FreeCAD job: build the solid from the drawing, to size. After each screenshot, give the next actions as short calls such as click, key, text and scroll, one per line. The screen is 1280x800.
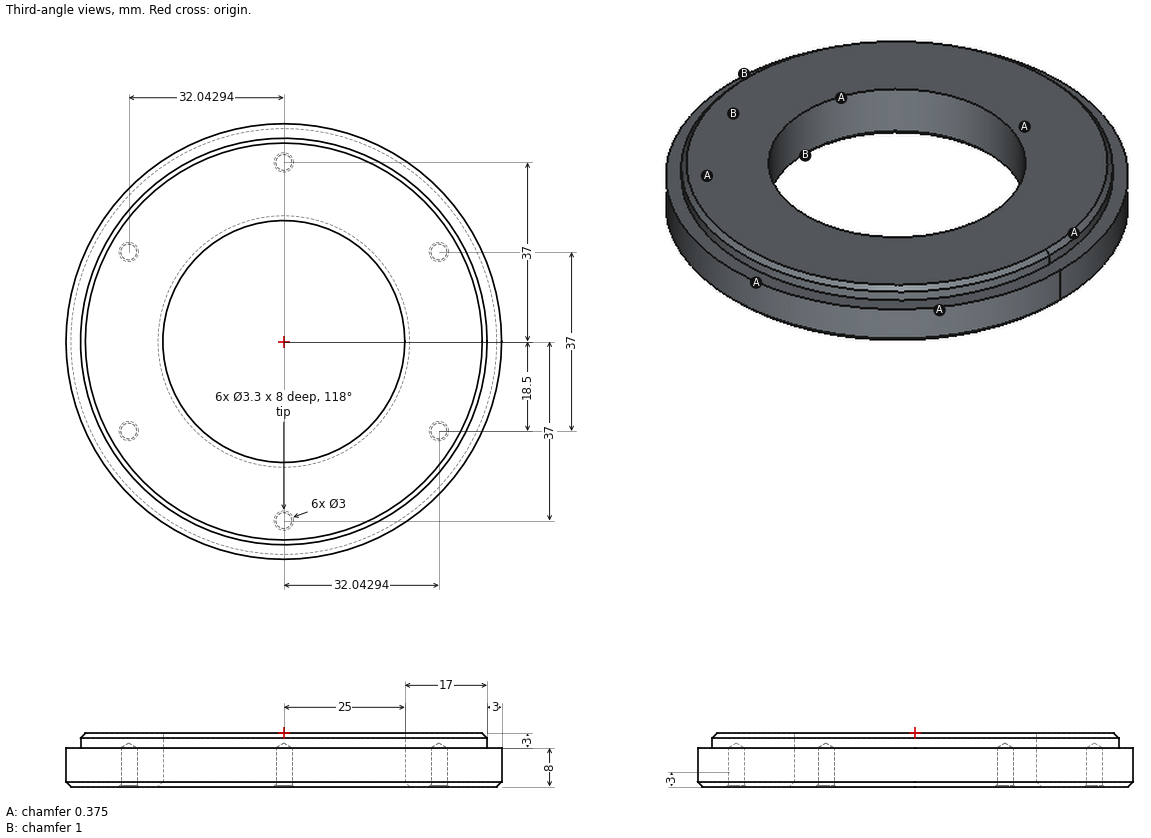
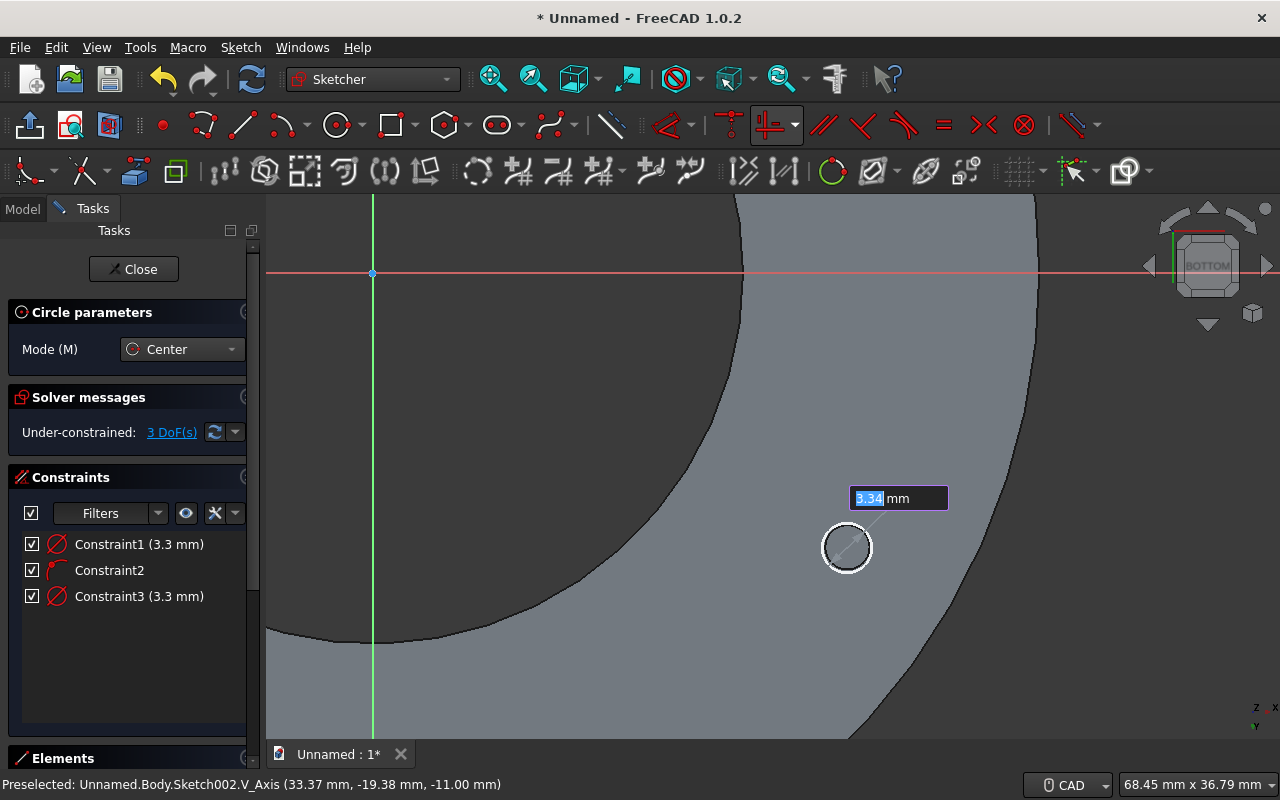
text(3.3)
key(Return)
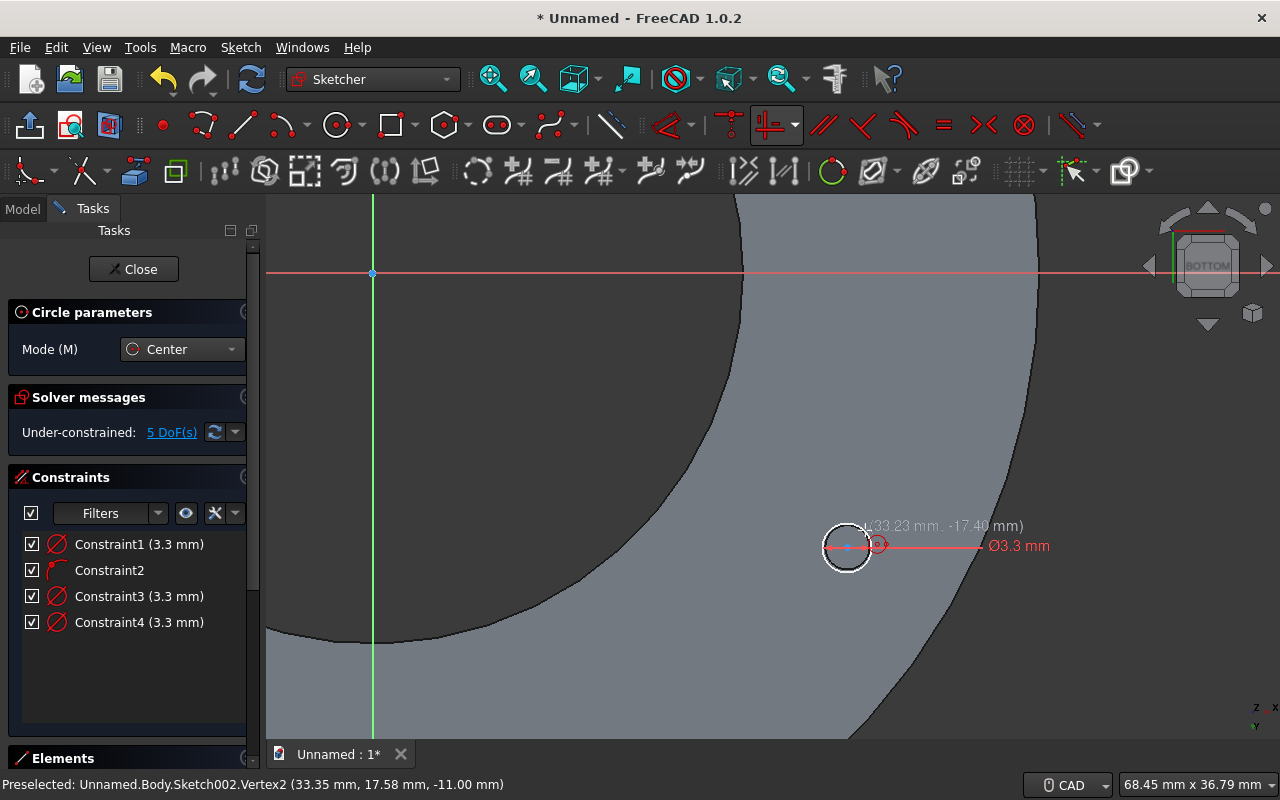
scroll(848, 550, down, 6)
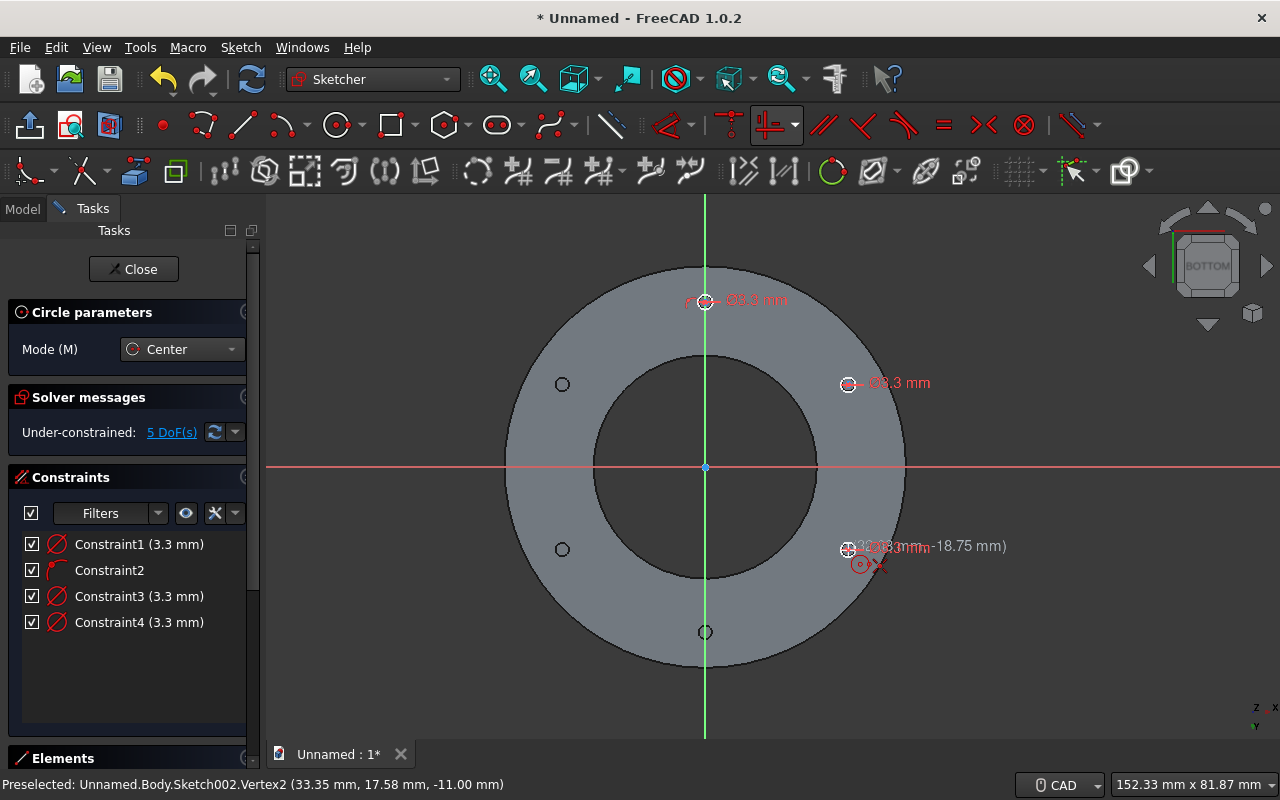
scroll(705, 632, up, 6)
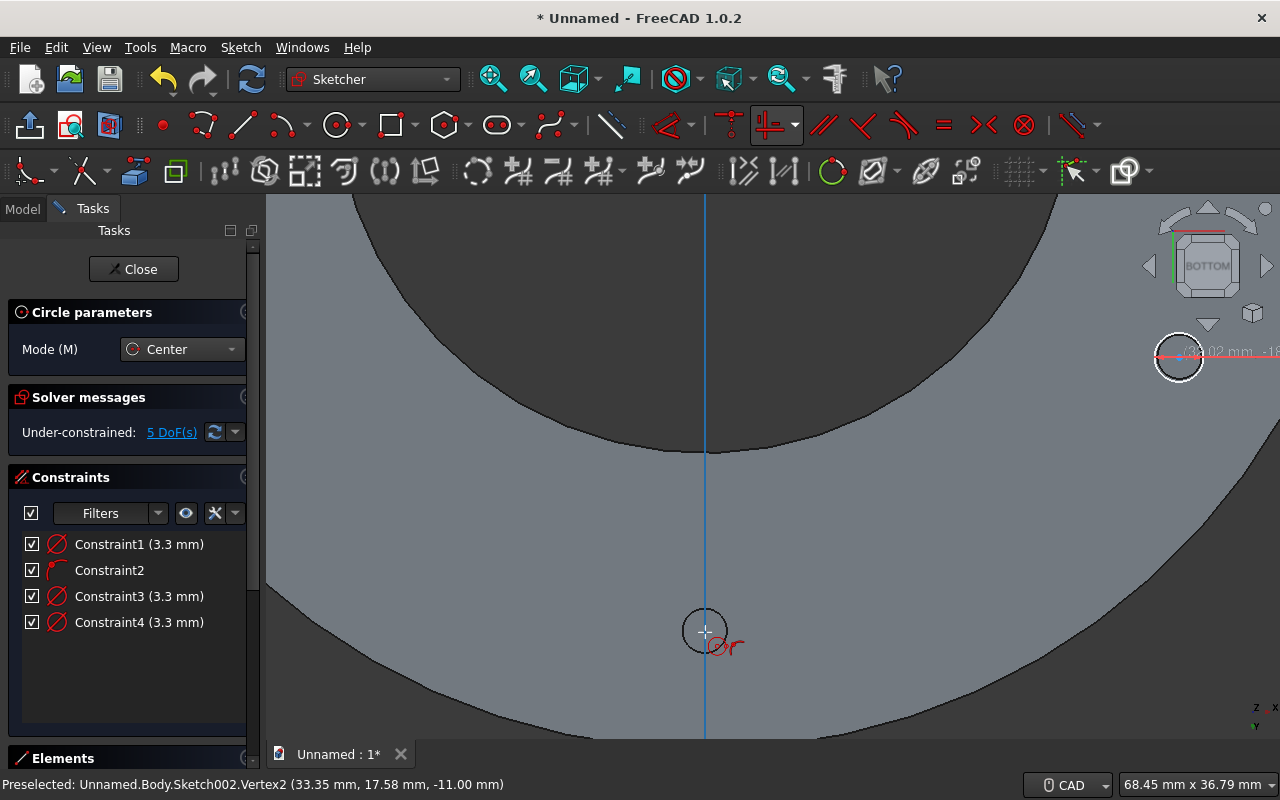
click(705, 631)
move(722, 614)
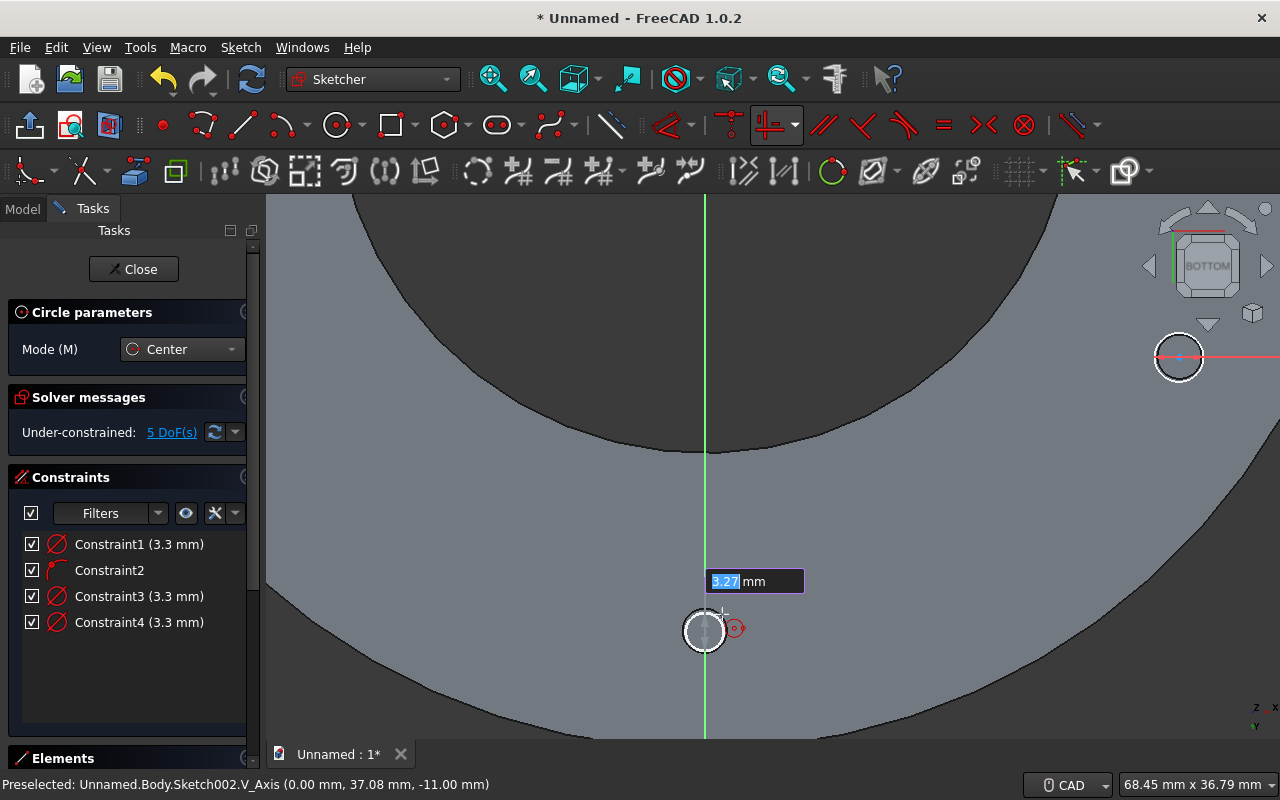
text(3.3)
key(Return)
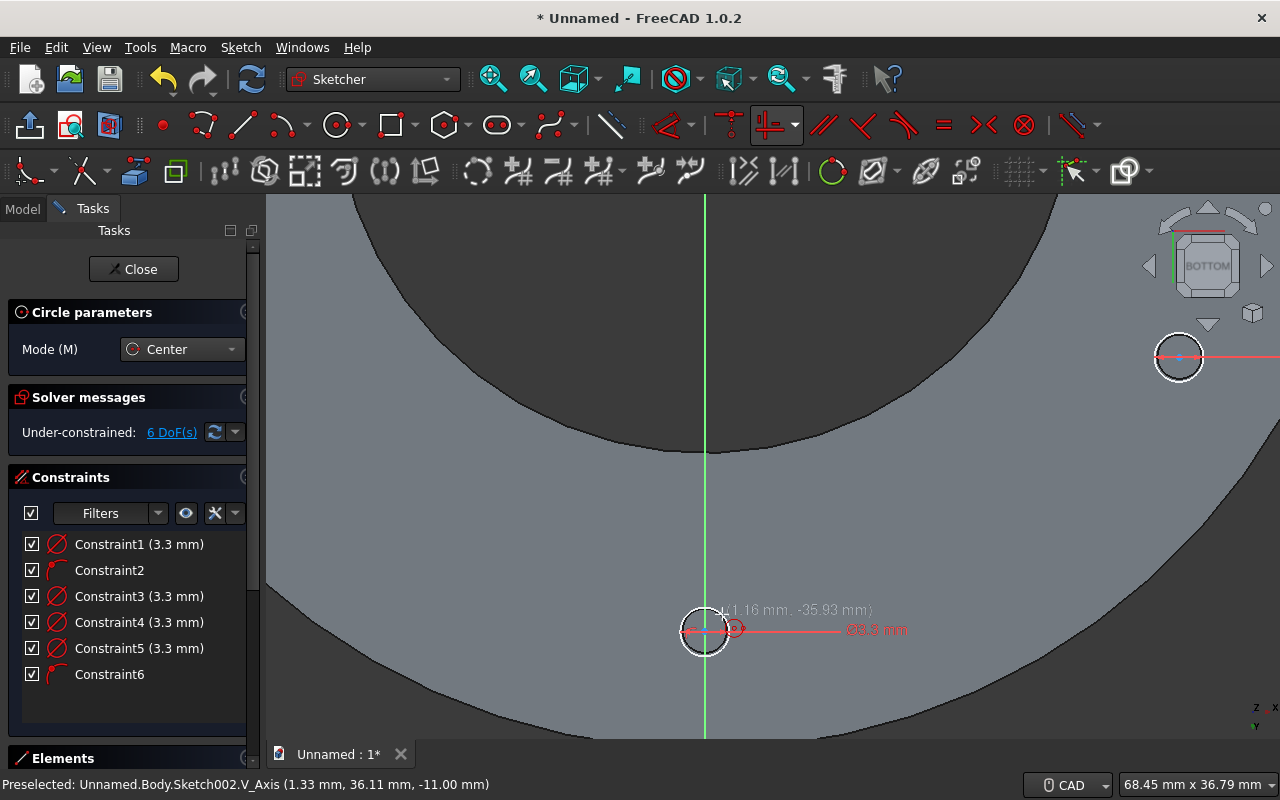
scroll(704, 632, down, 6)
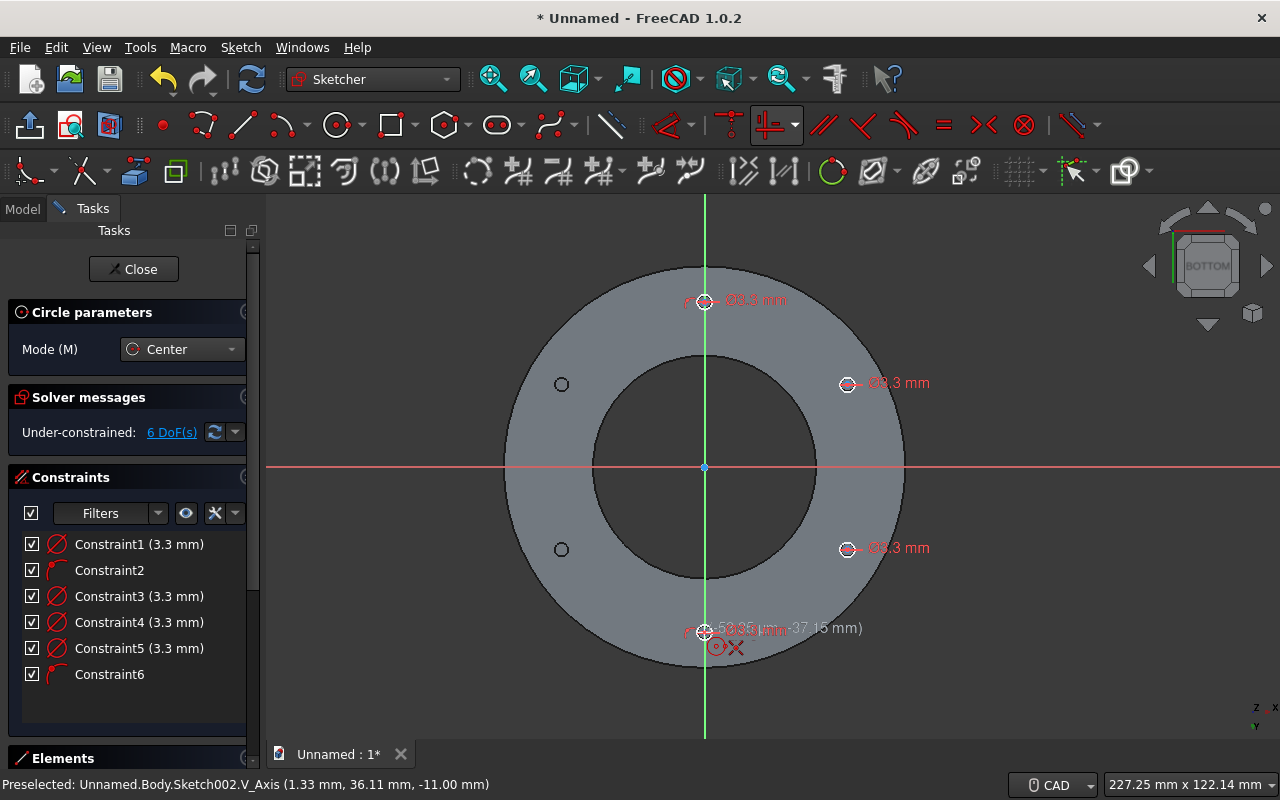
scroll(562, 385, up, 6)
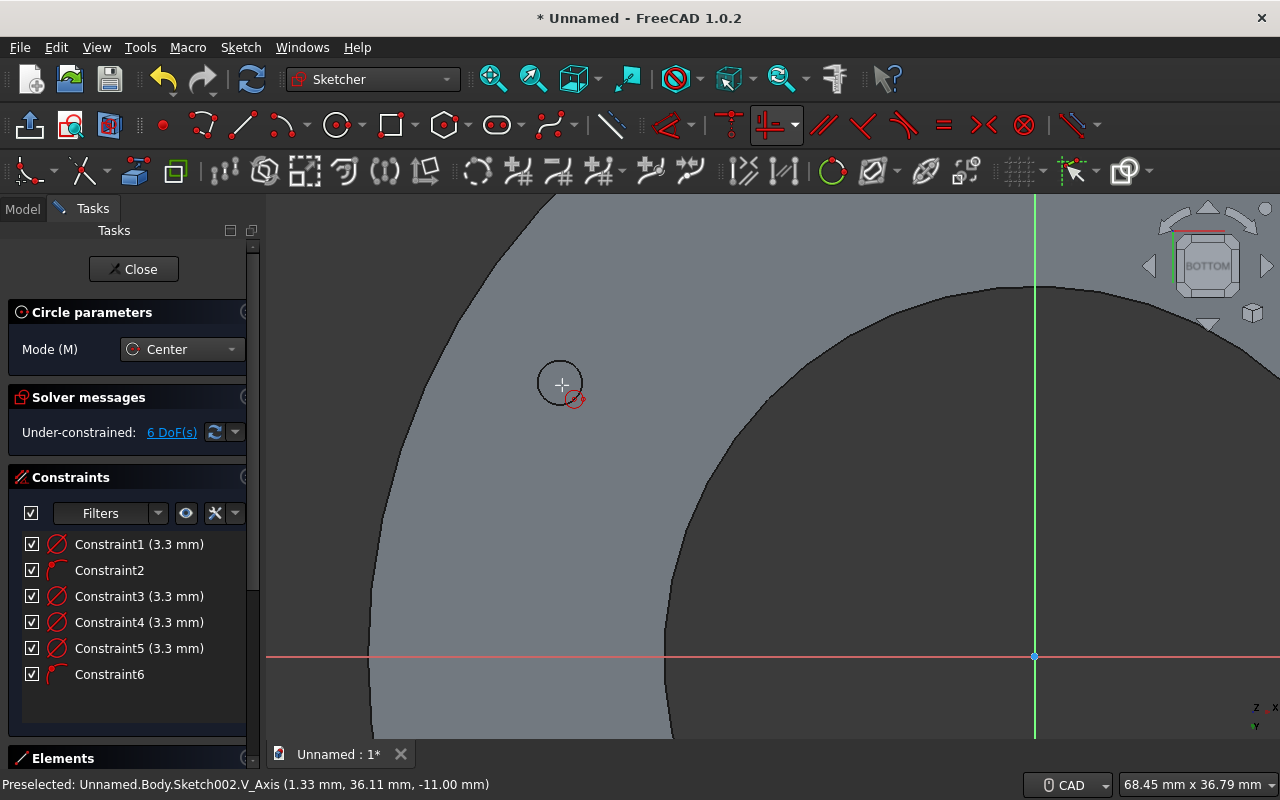
click(560, 383)
move(577, 365)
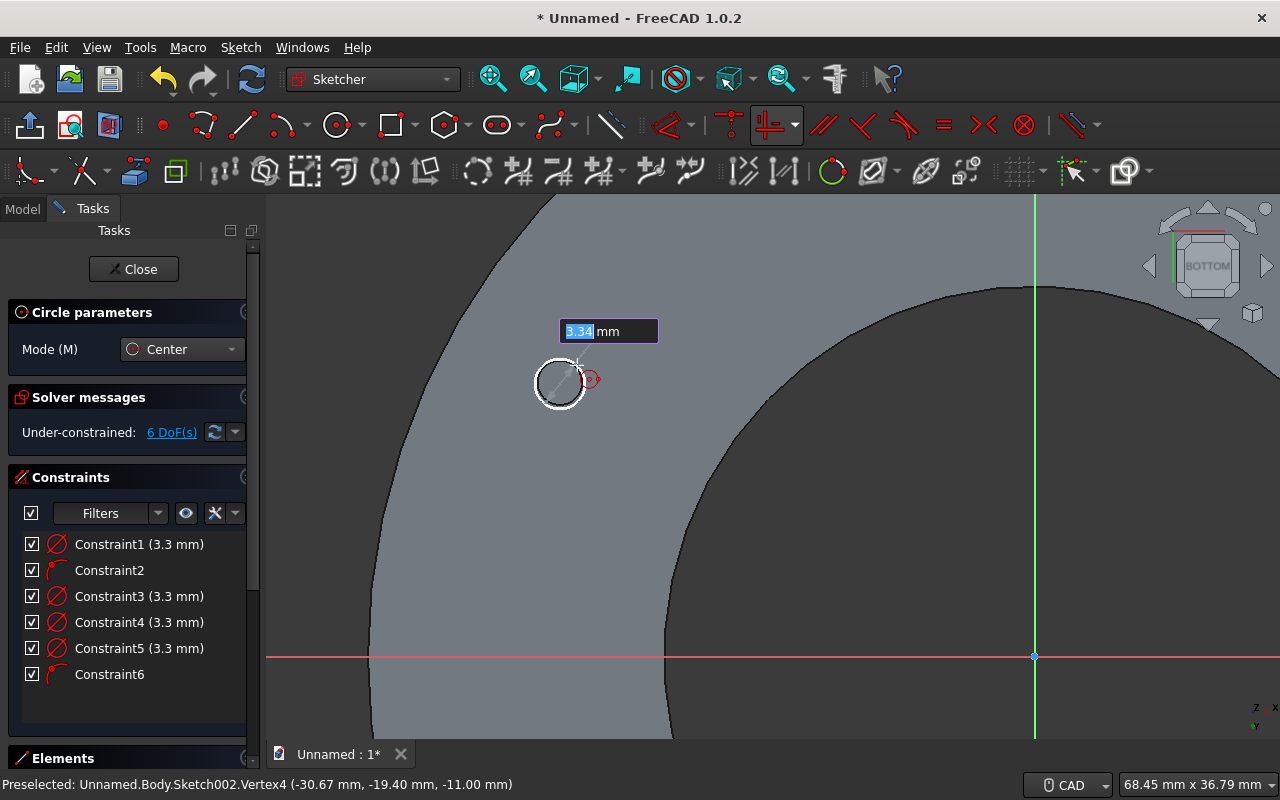
text(3.3)
key(Return)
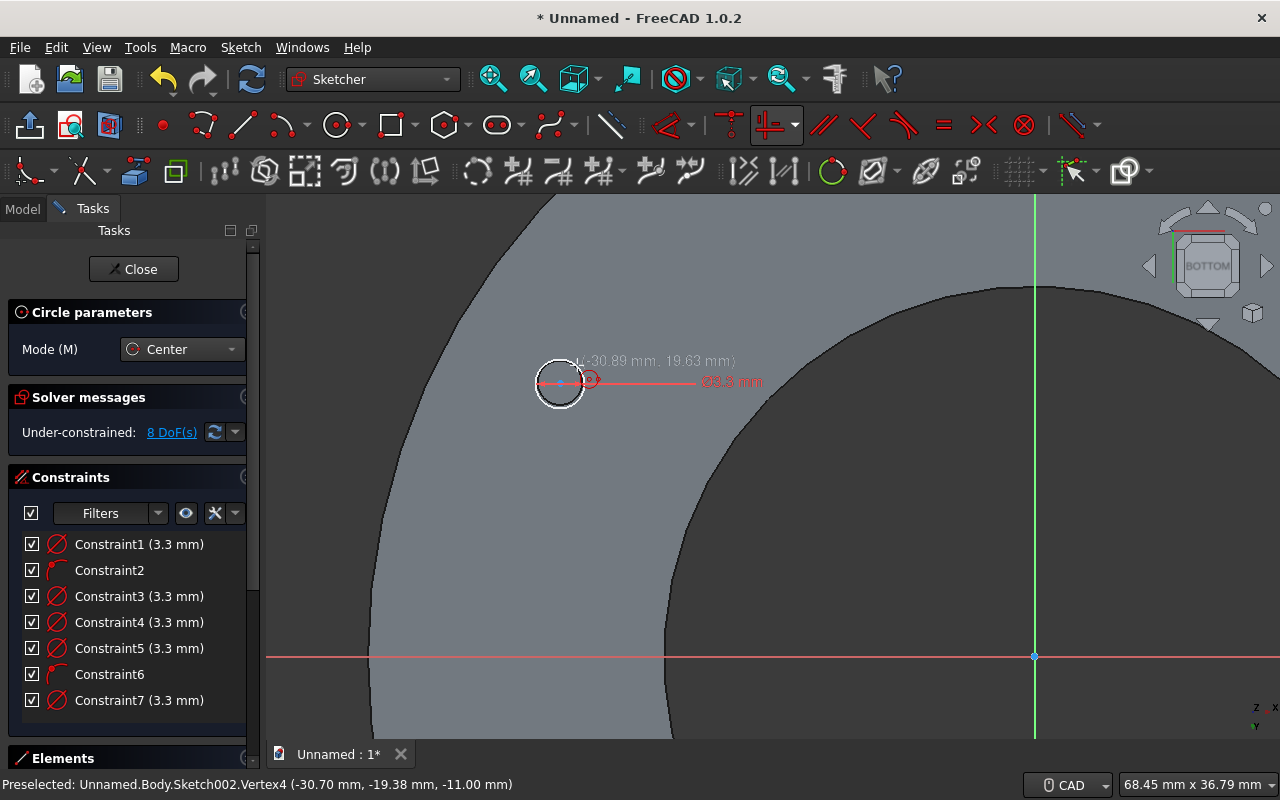
scroll(562, 384, down, 6)